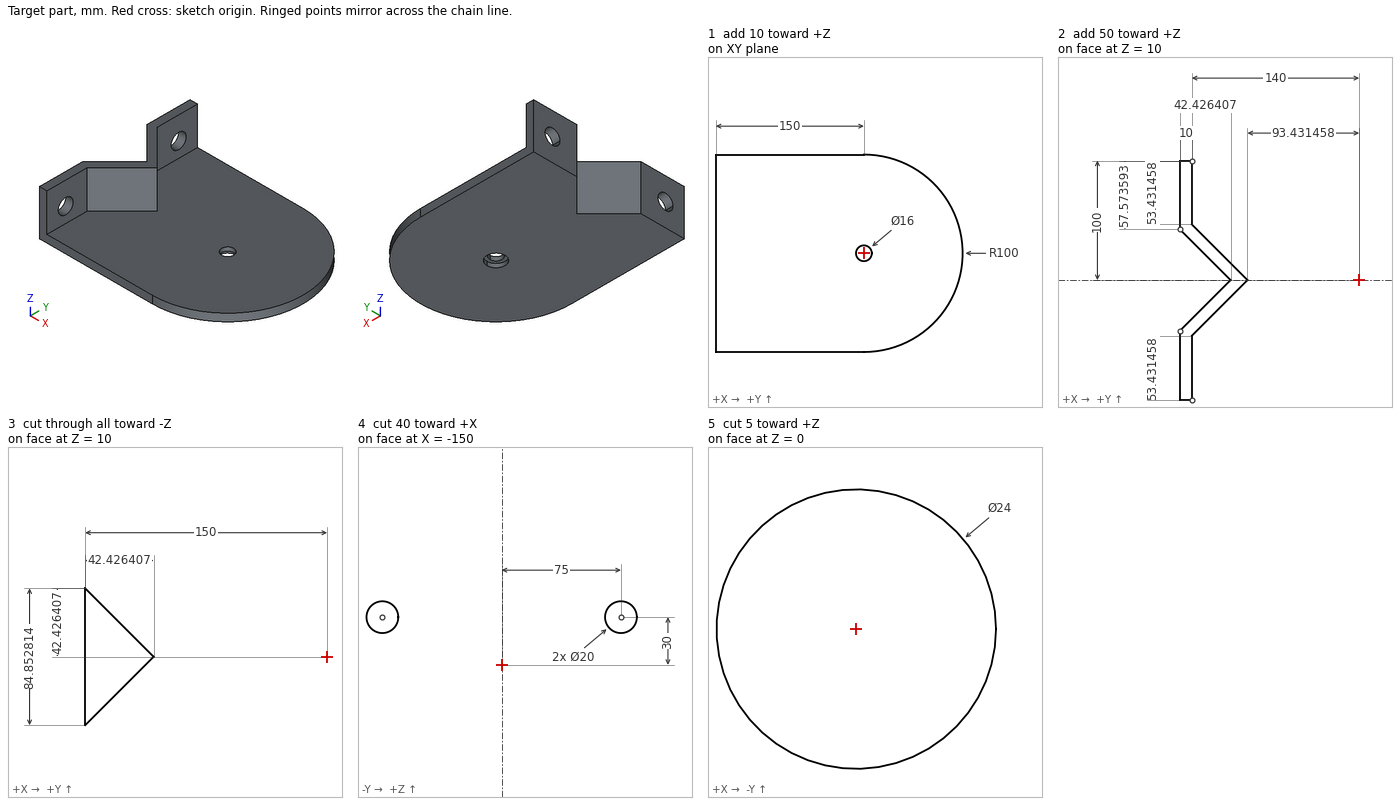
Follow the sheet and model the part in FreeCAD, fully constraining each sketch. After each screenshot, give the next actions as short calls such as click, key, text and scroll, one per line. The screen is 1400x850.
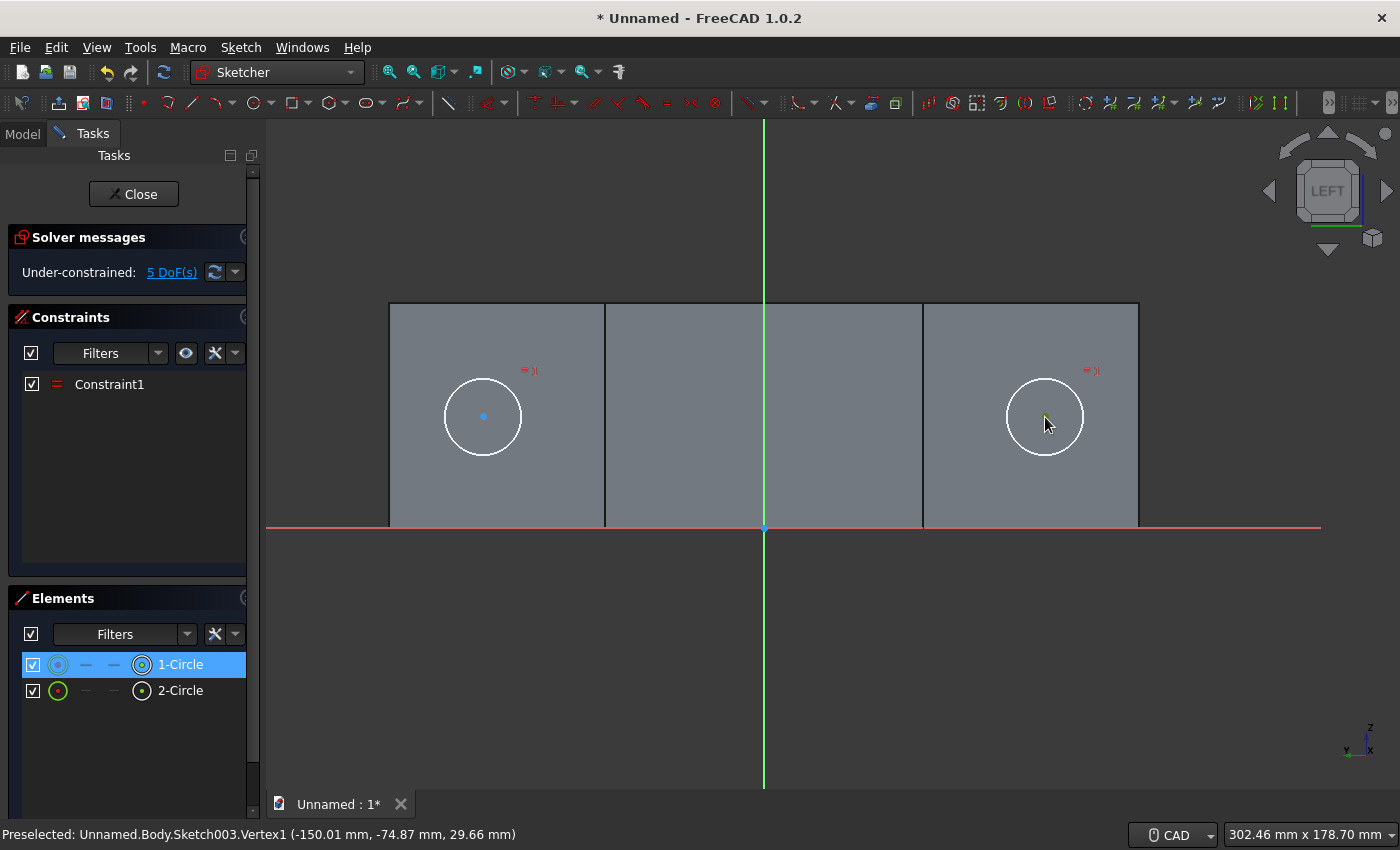
click(483, 417)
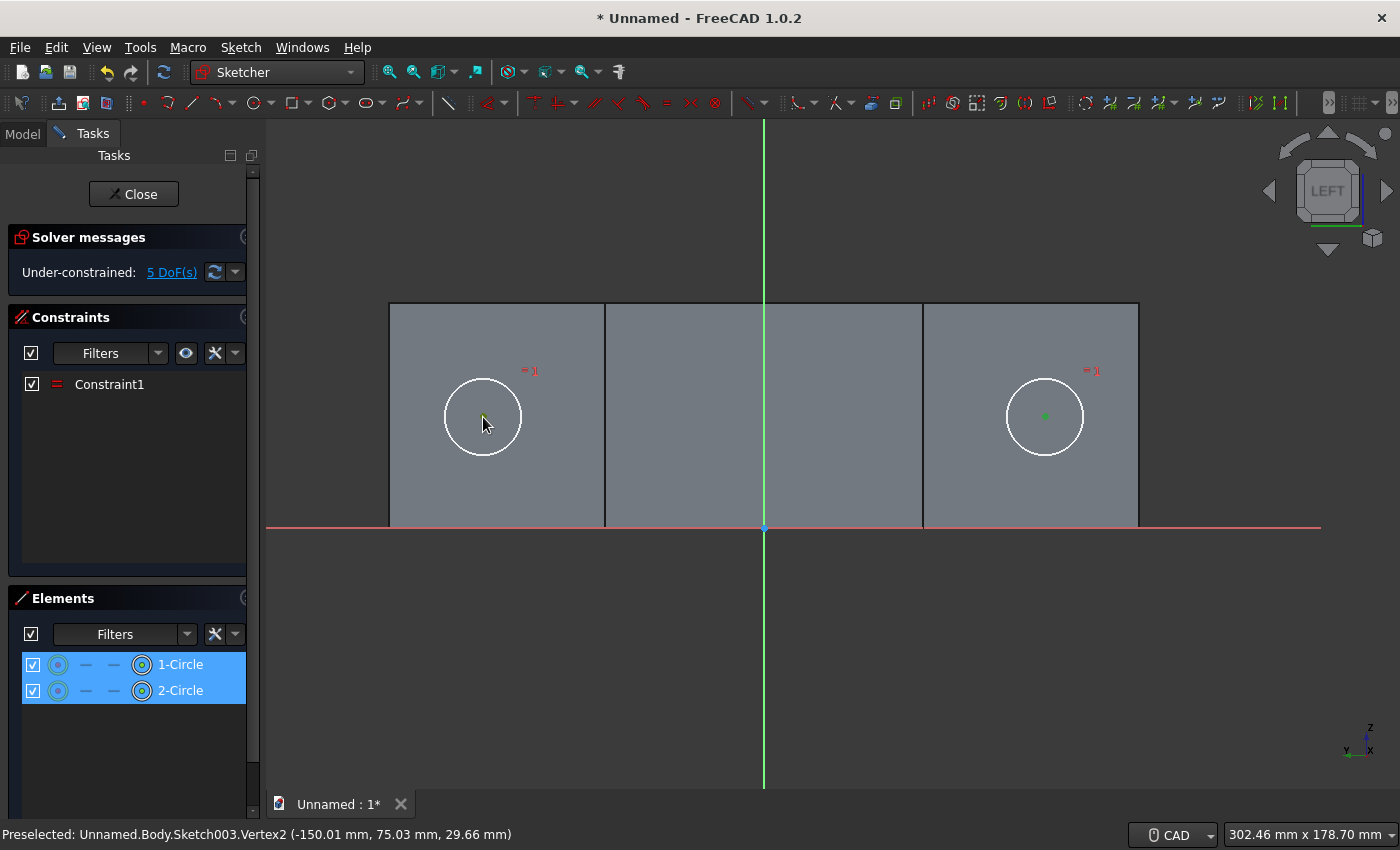
click(764, 717)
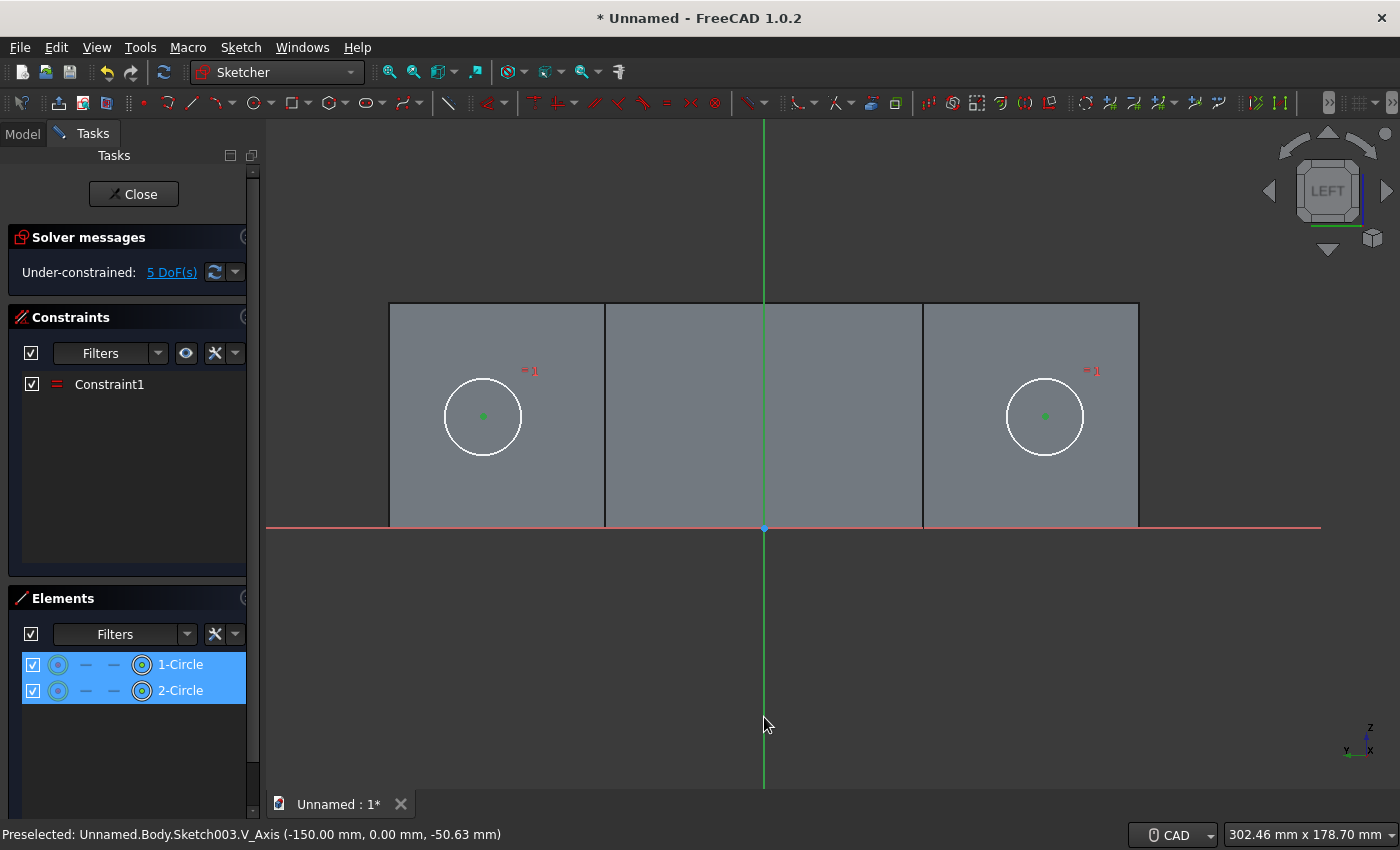
click(692, 104)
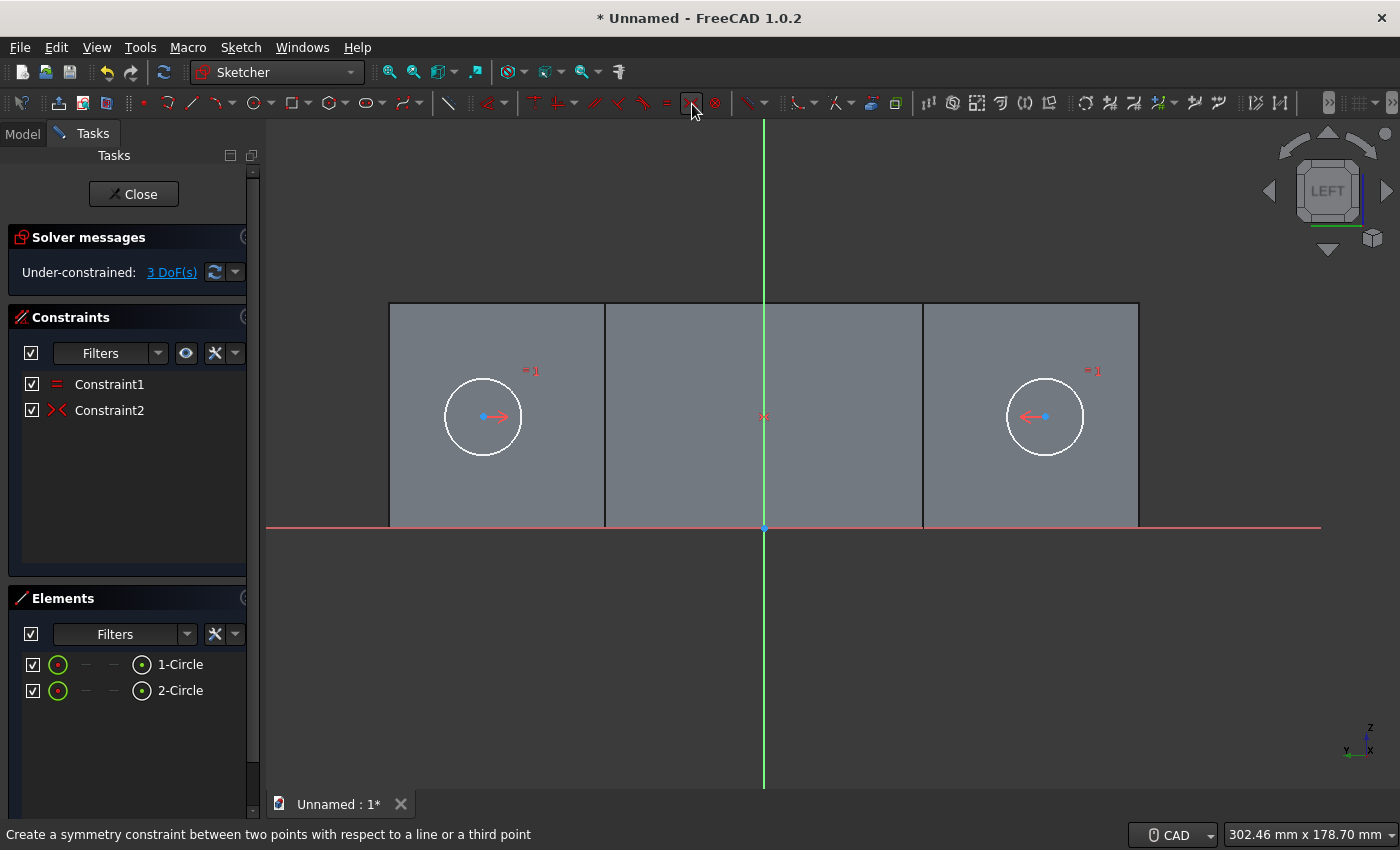
click(488, 104)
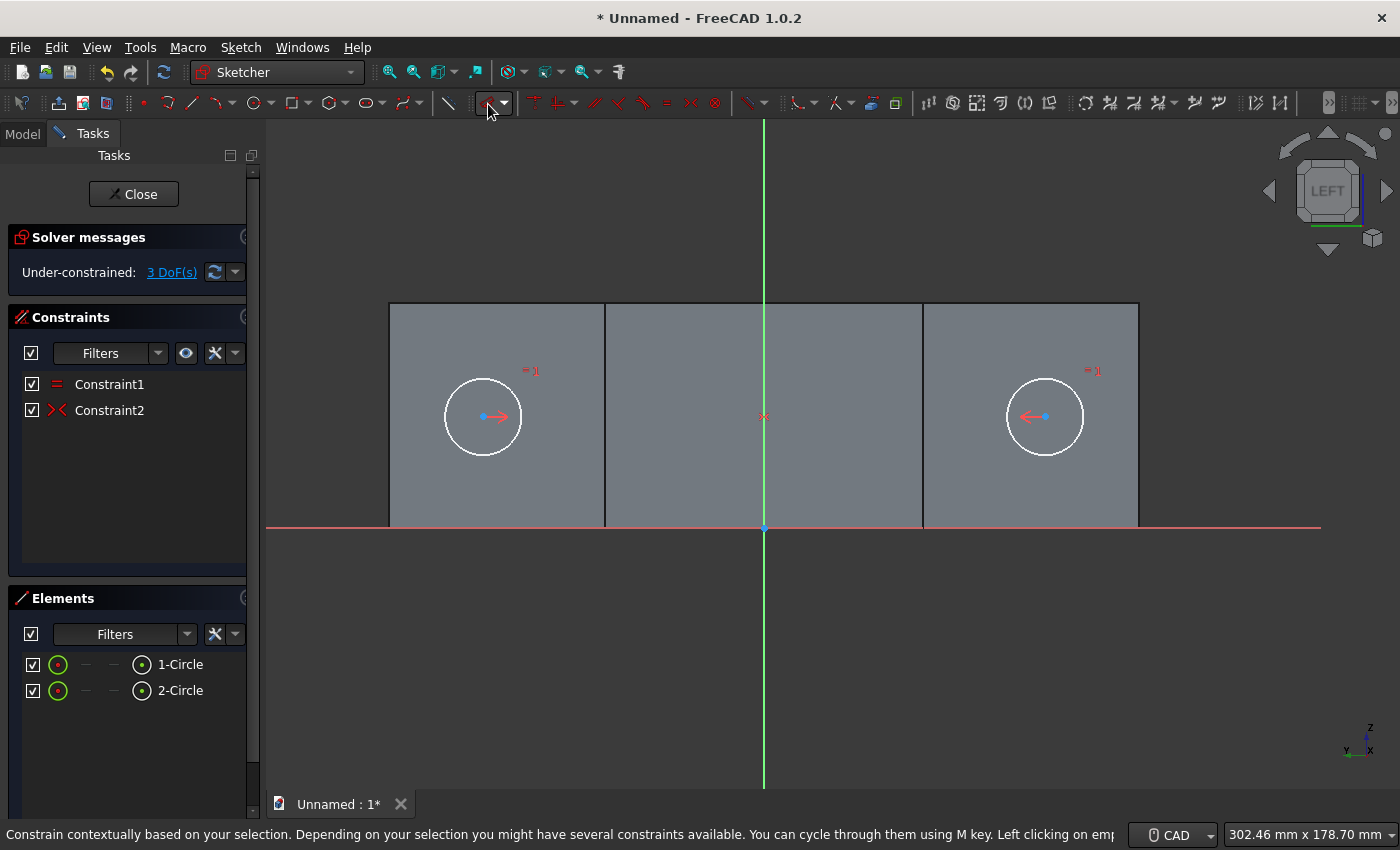
click(1072, 390)
click(1094, 367)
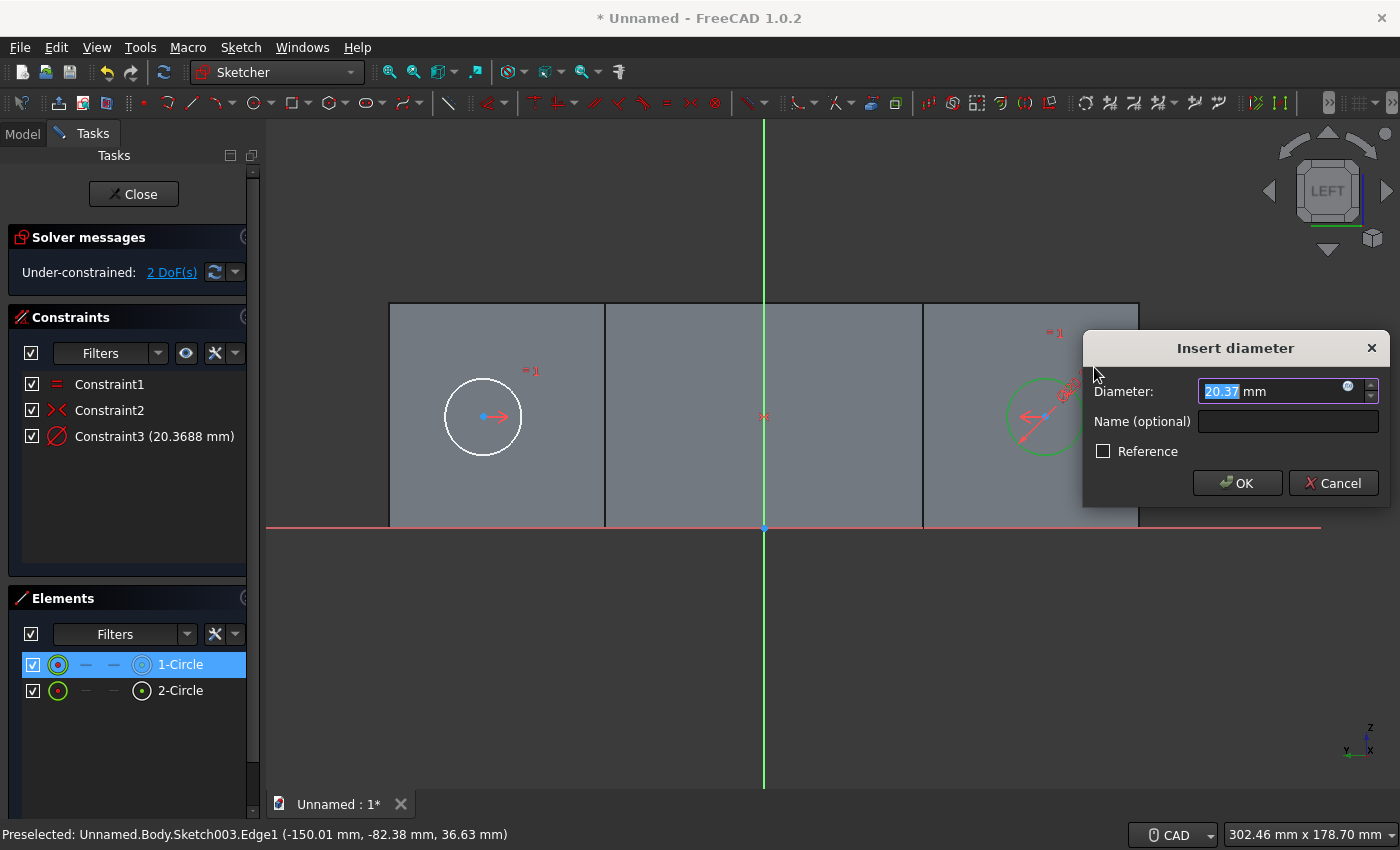
text(20)
key(Return)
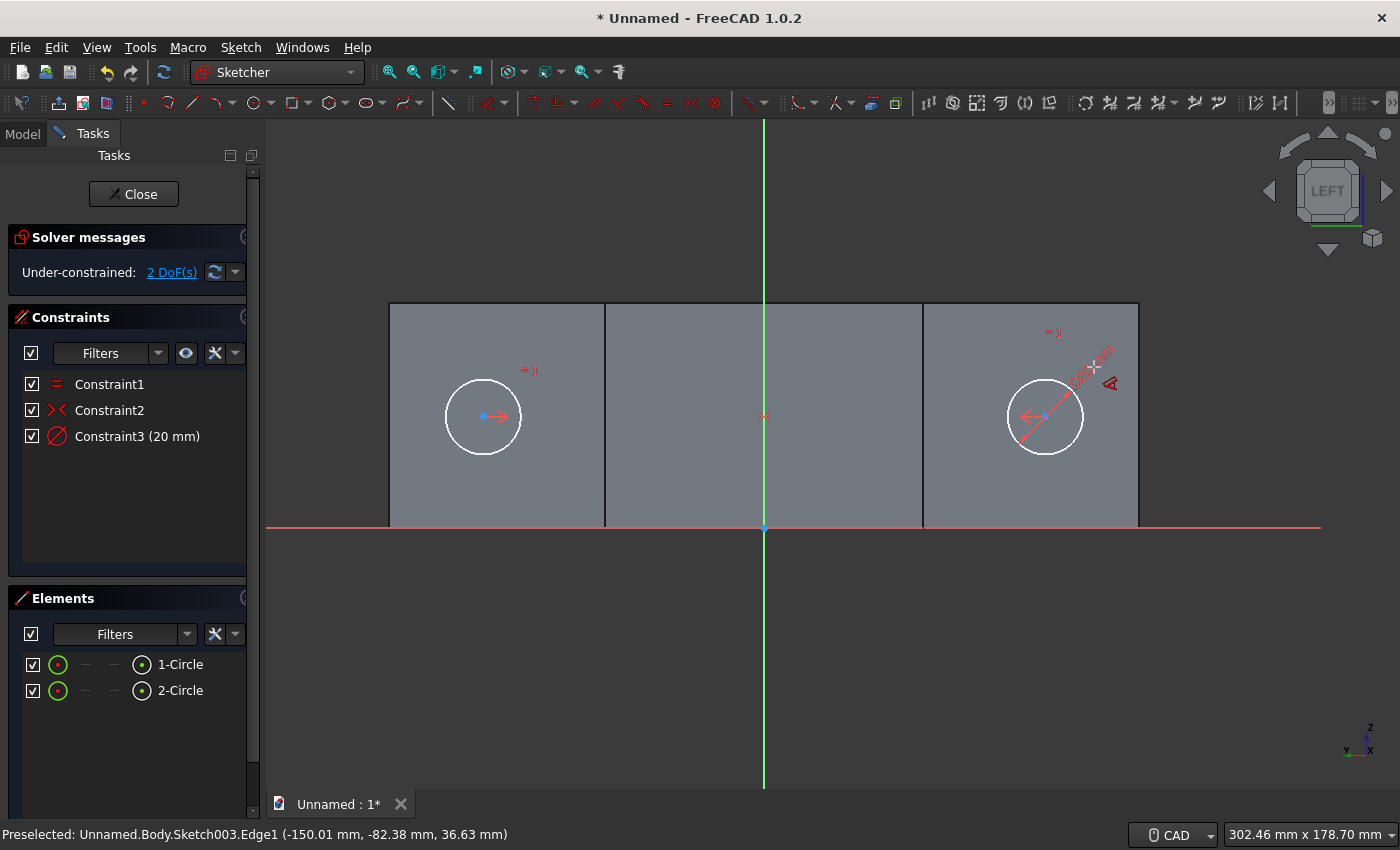
click(1045, 417)
click(905, 562)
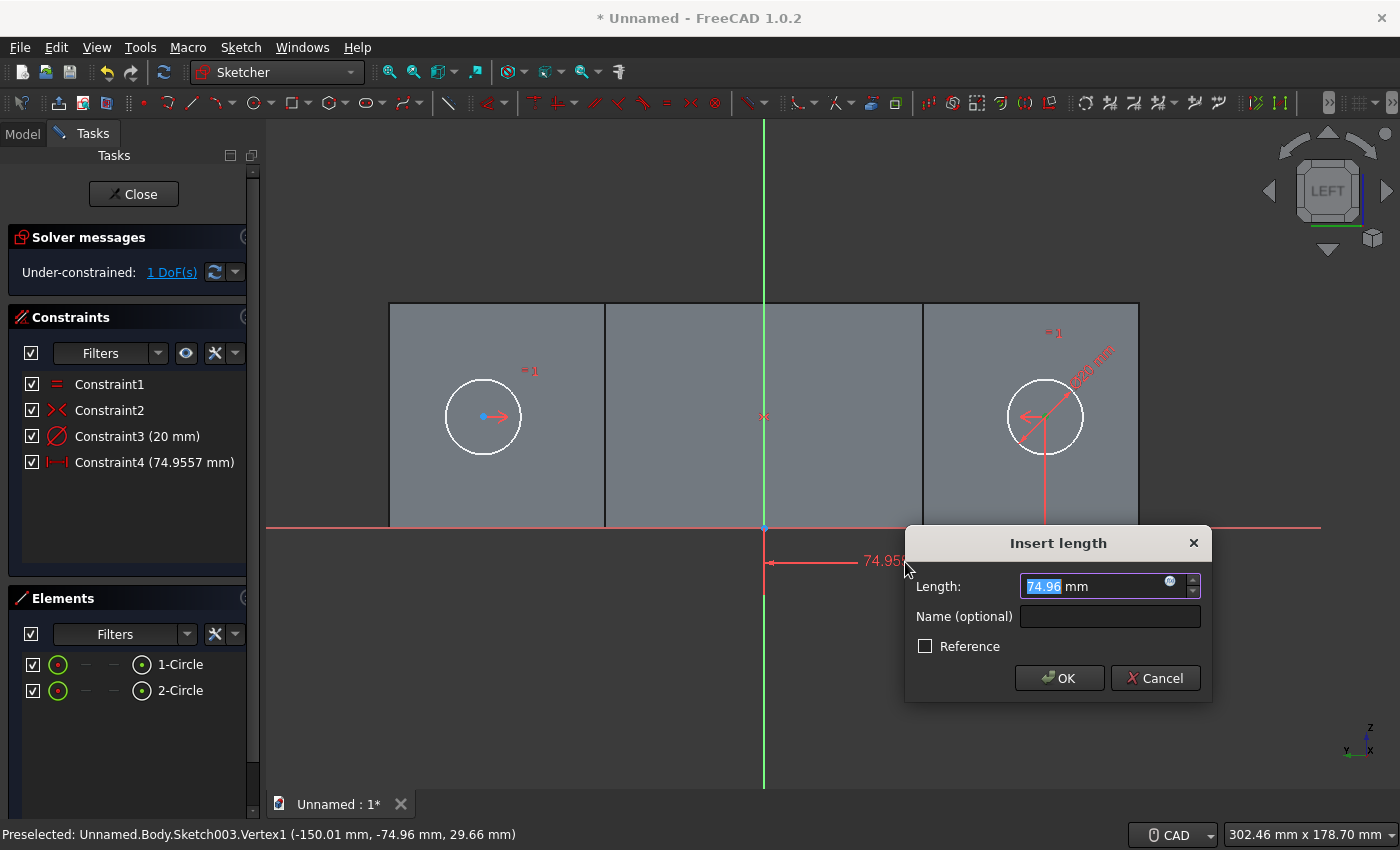
text(75)
key(Return)